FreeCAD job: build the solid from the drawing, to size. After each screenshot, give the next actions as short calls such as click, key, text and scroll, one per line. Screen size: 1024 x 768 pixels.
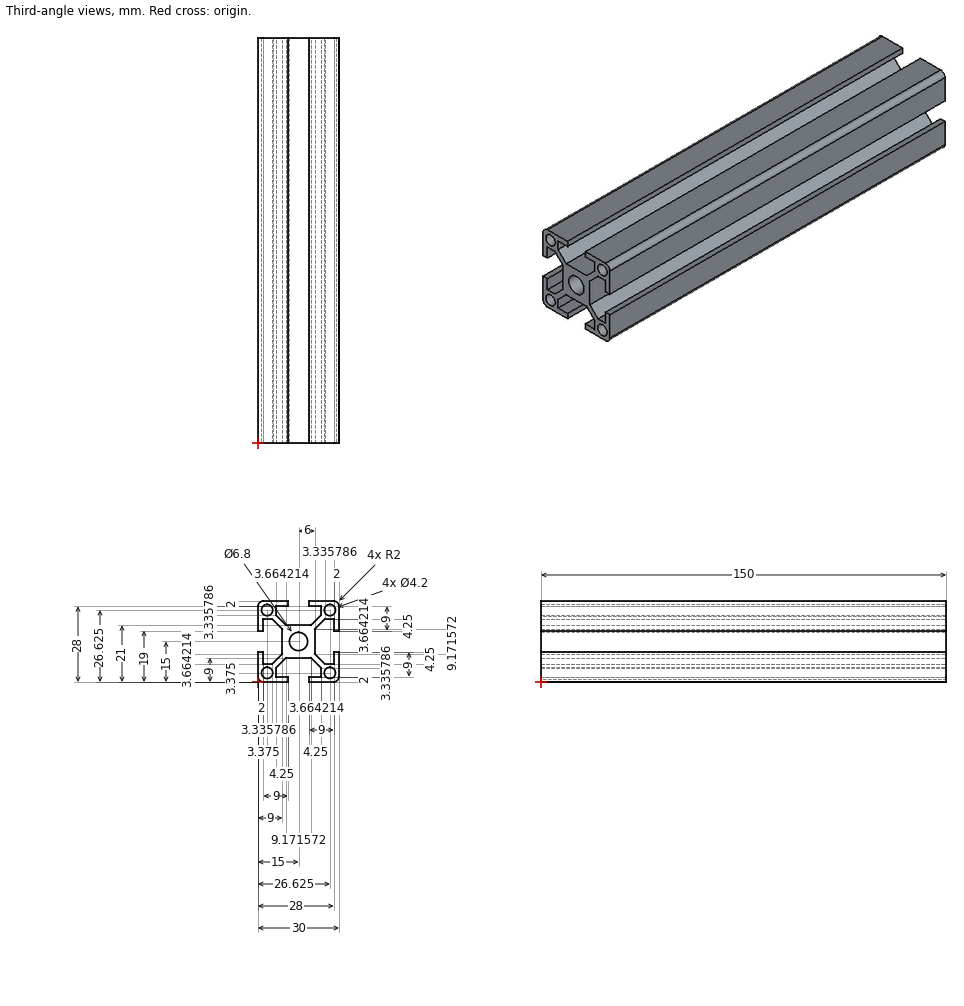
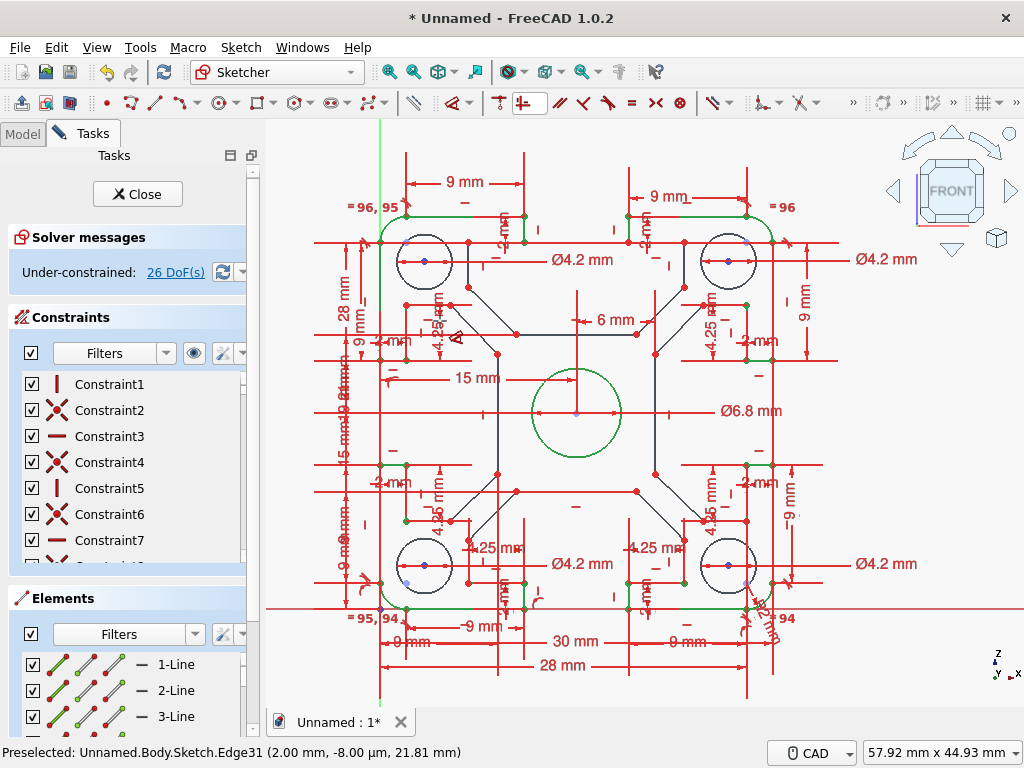
click(507, 243)
click(496, 277)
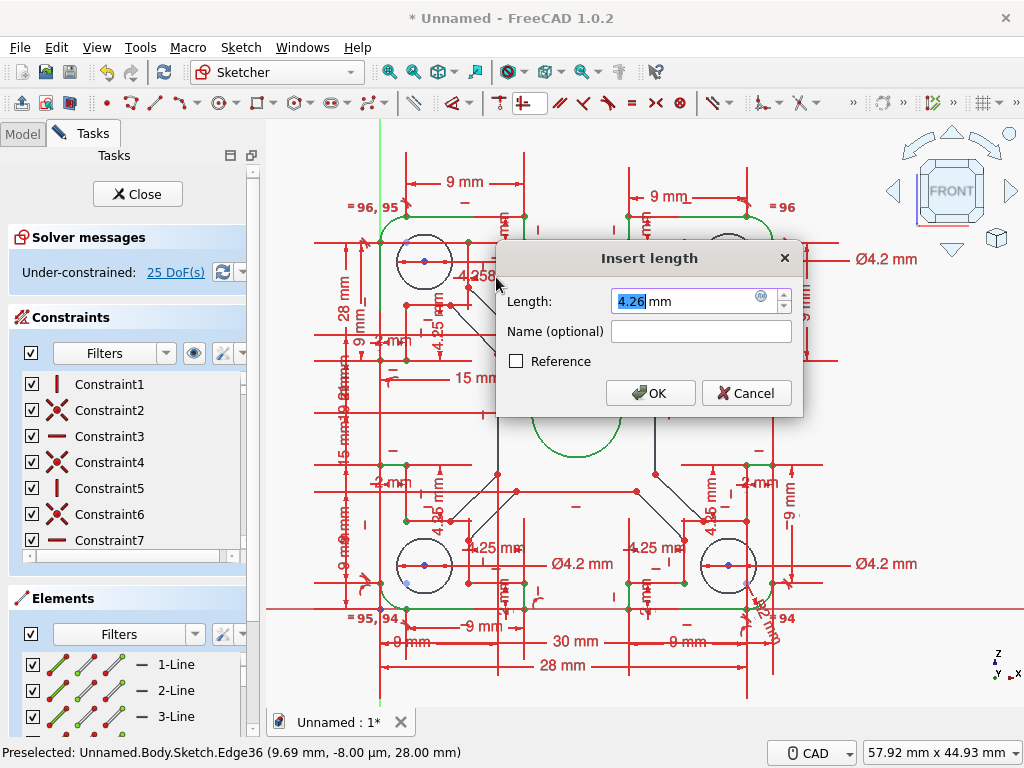
text(4.25)
key(Return)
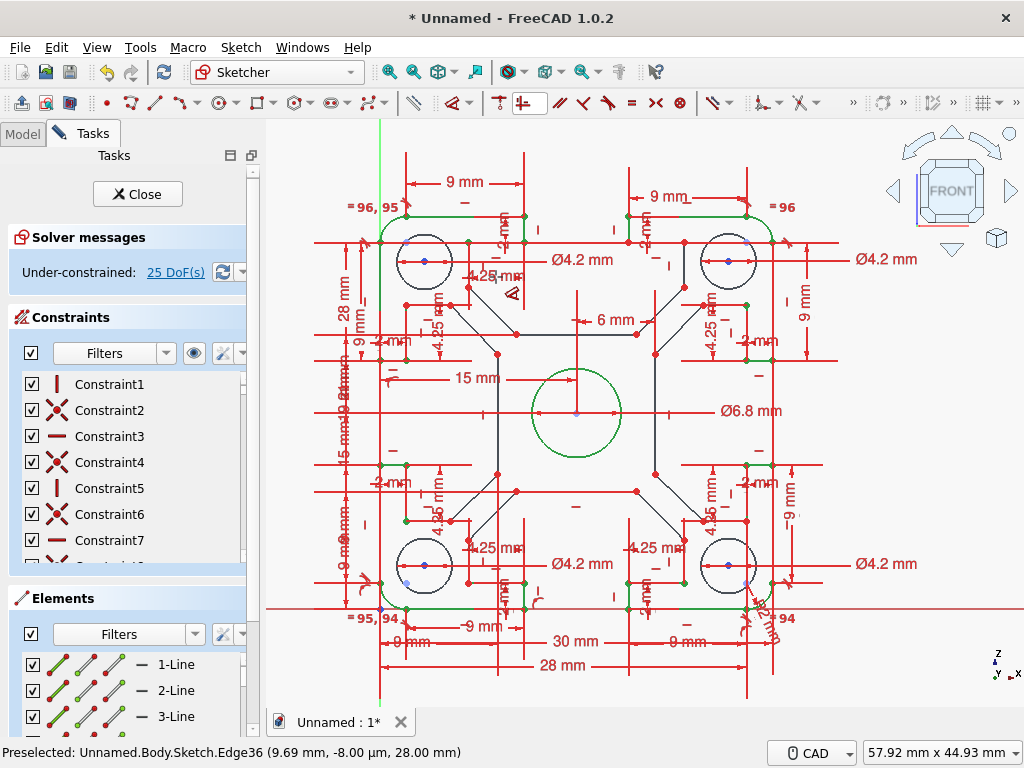
click(668, 243)
click(657, 277)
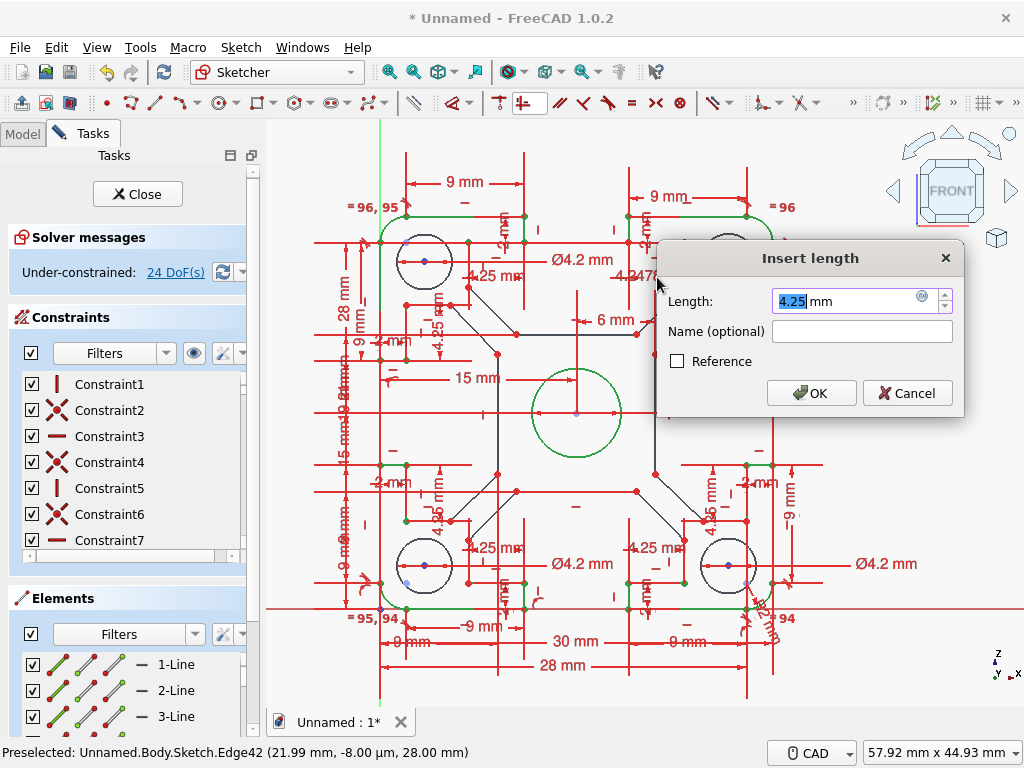
text(4.25)
key(Return)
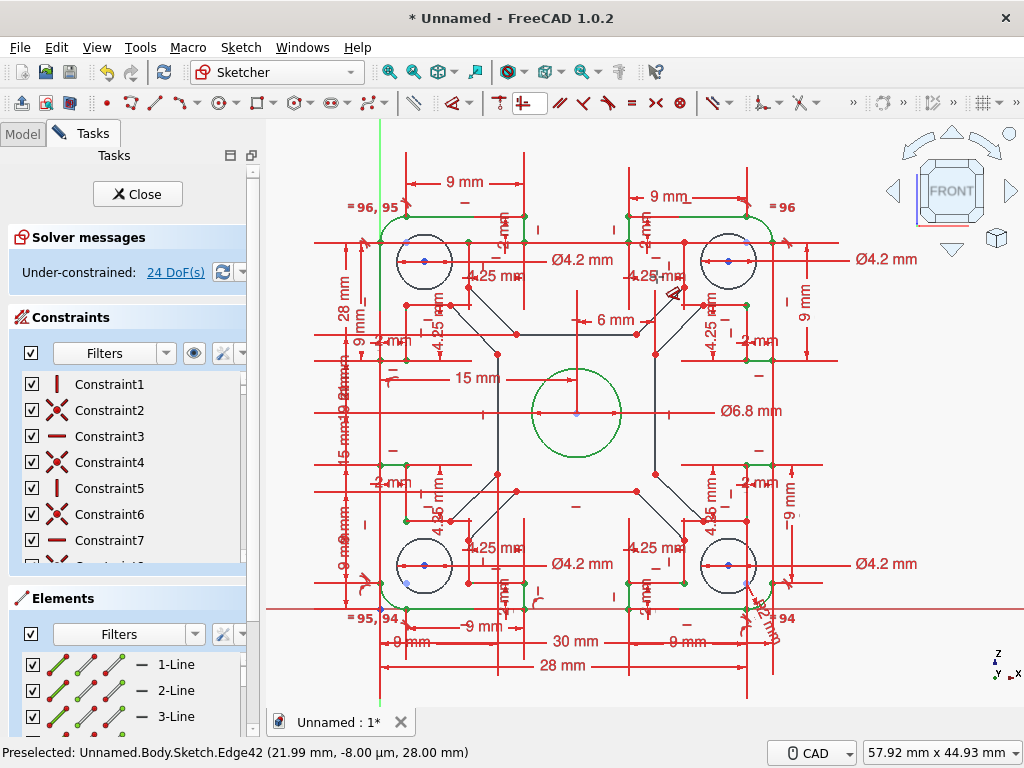
click(425, 262)
click(402, 667)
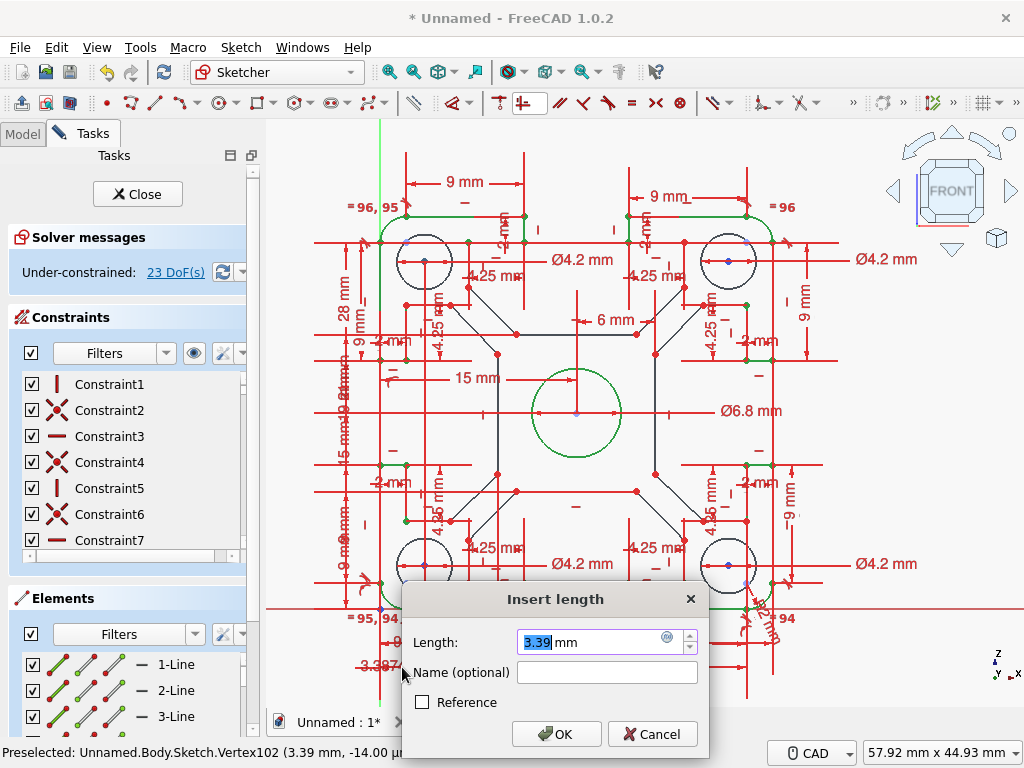
text(3.375)
key(Return)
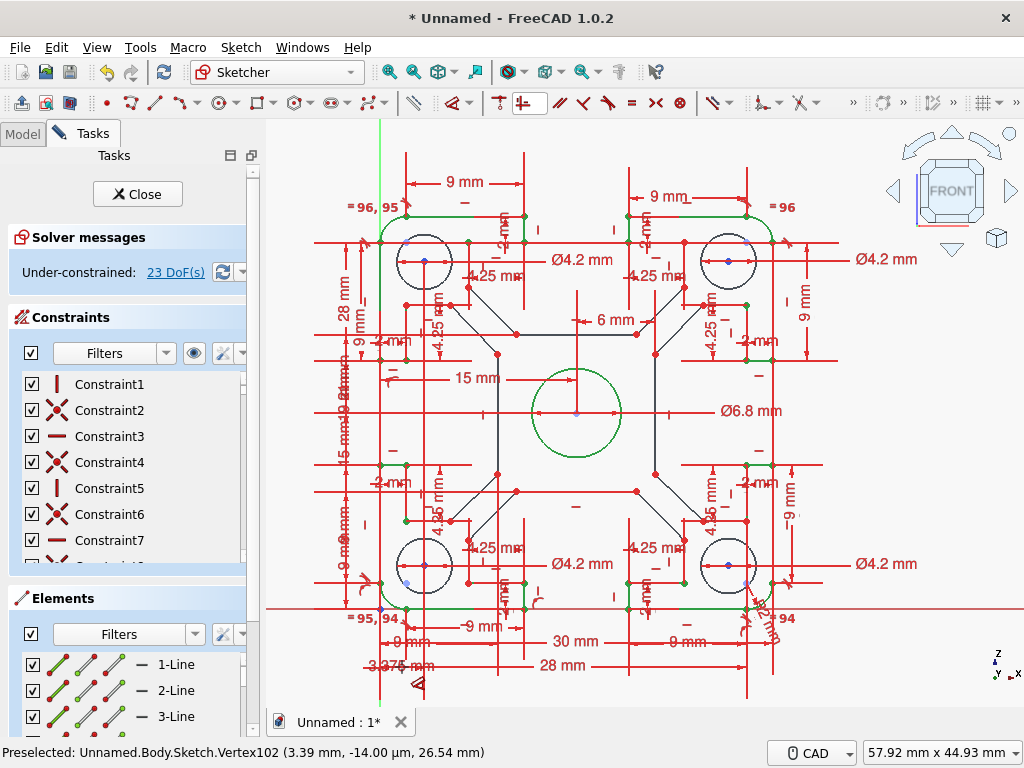
click(729, 566)
click(346, 588)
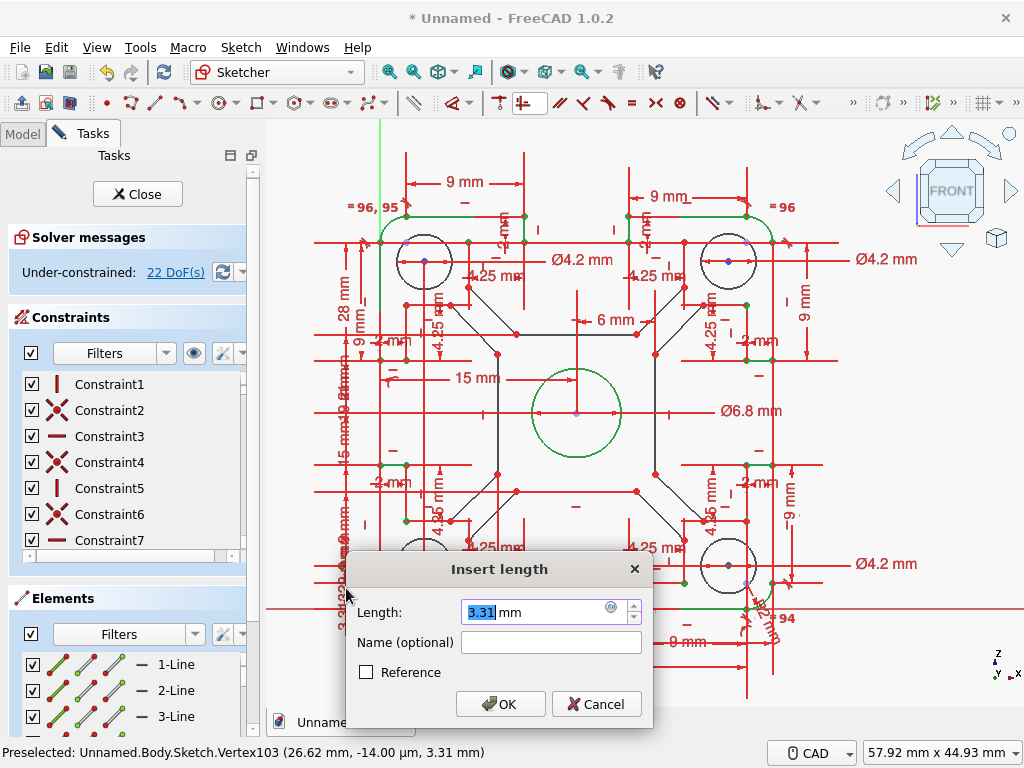
text(3.375)
key(Return)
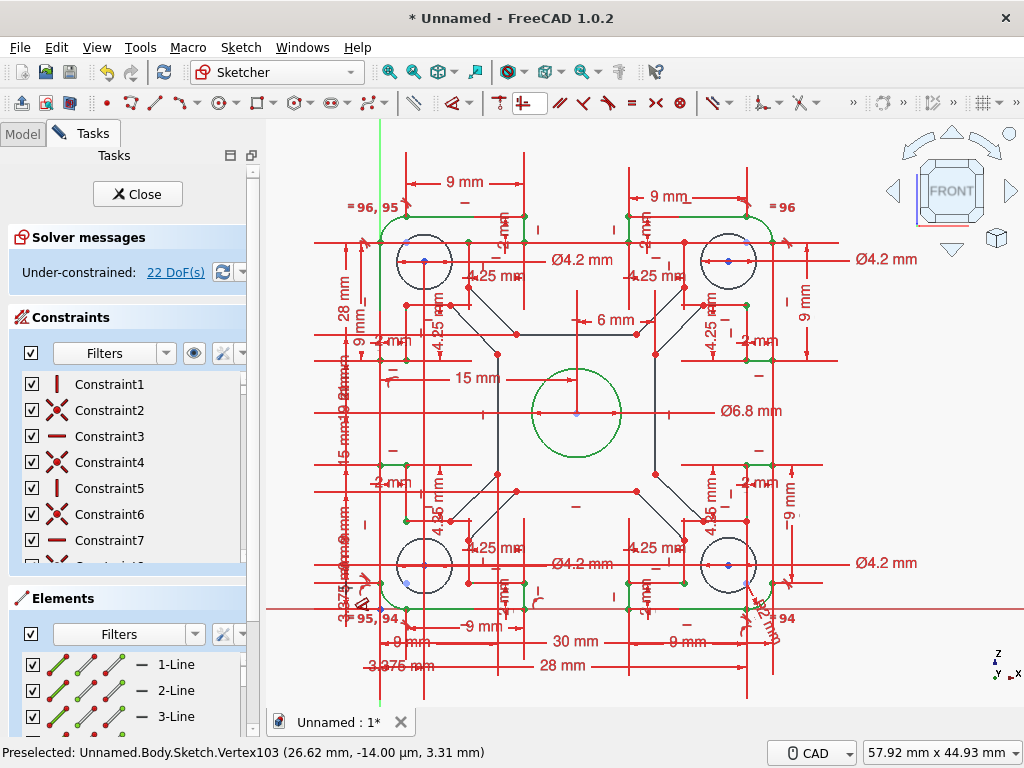
click(425, 566)
click(418, 436)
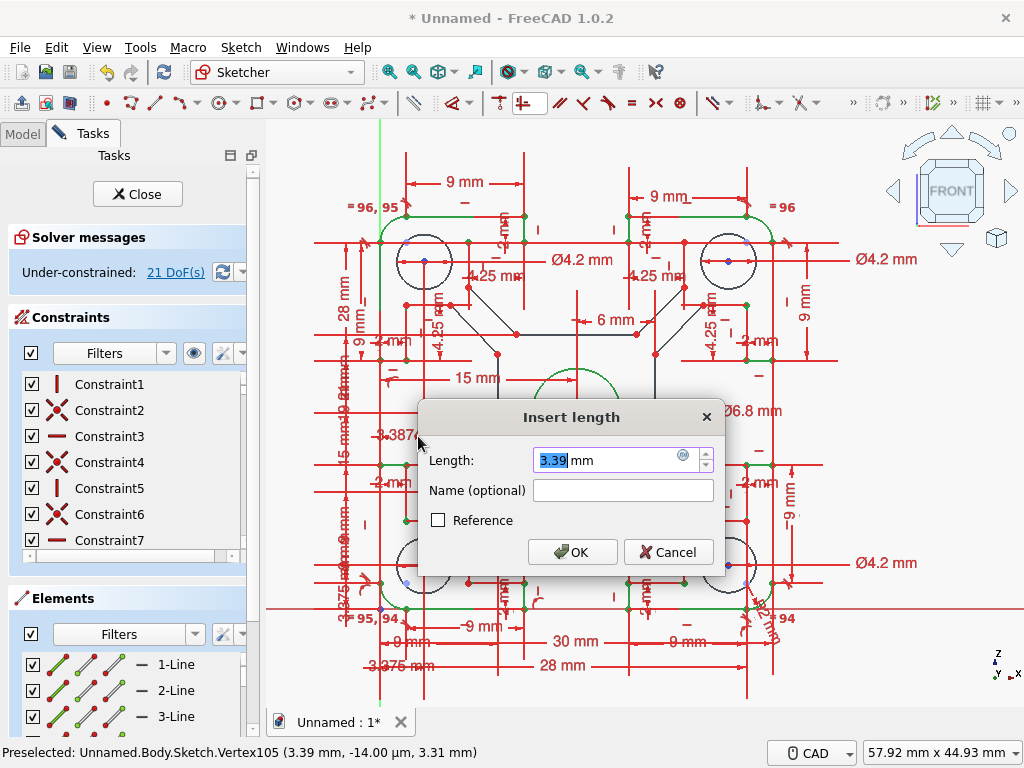
text(3.375)
key(Return)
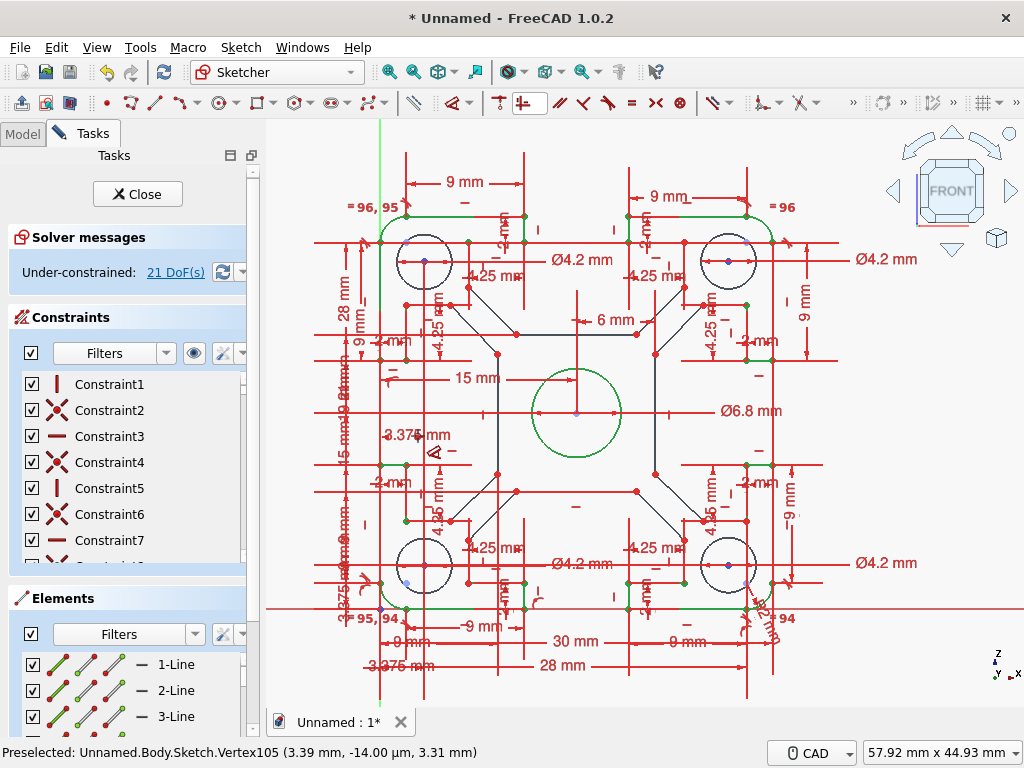
click(424, 566)
click(554, 573)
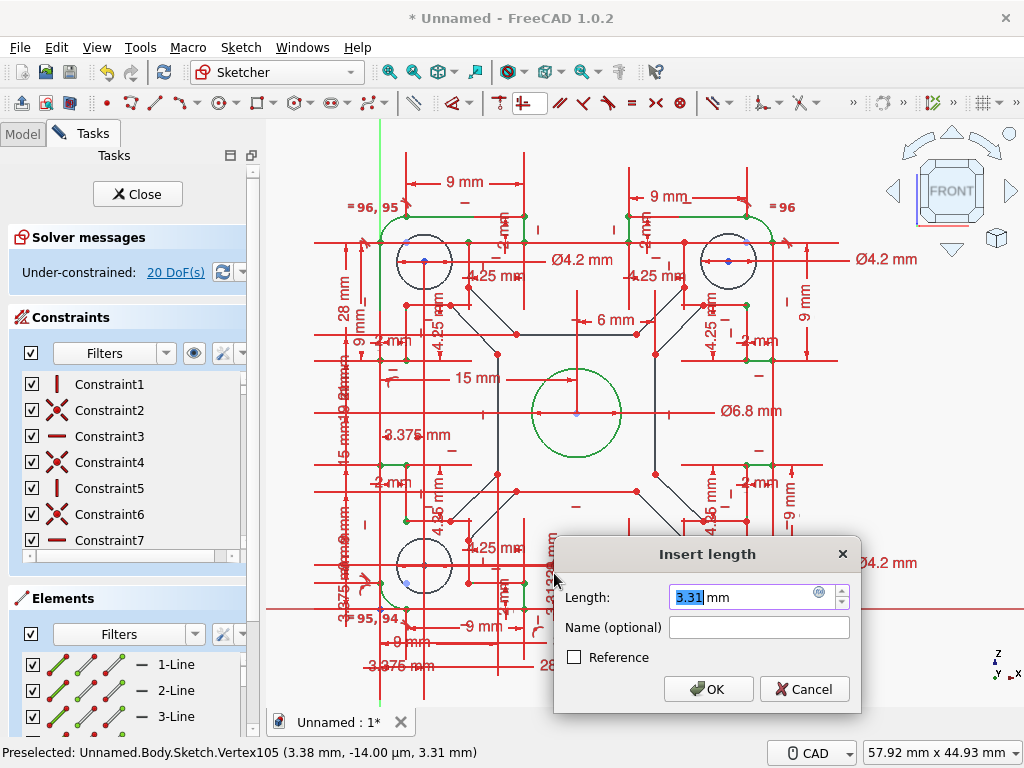
text(3.375)
key(Return)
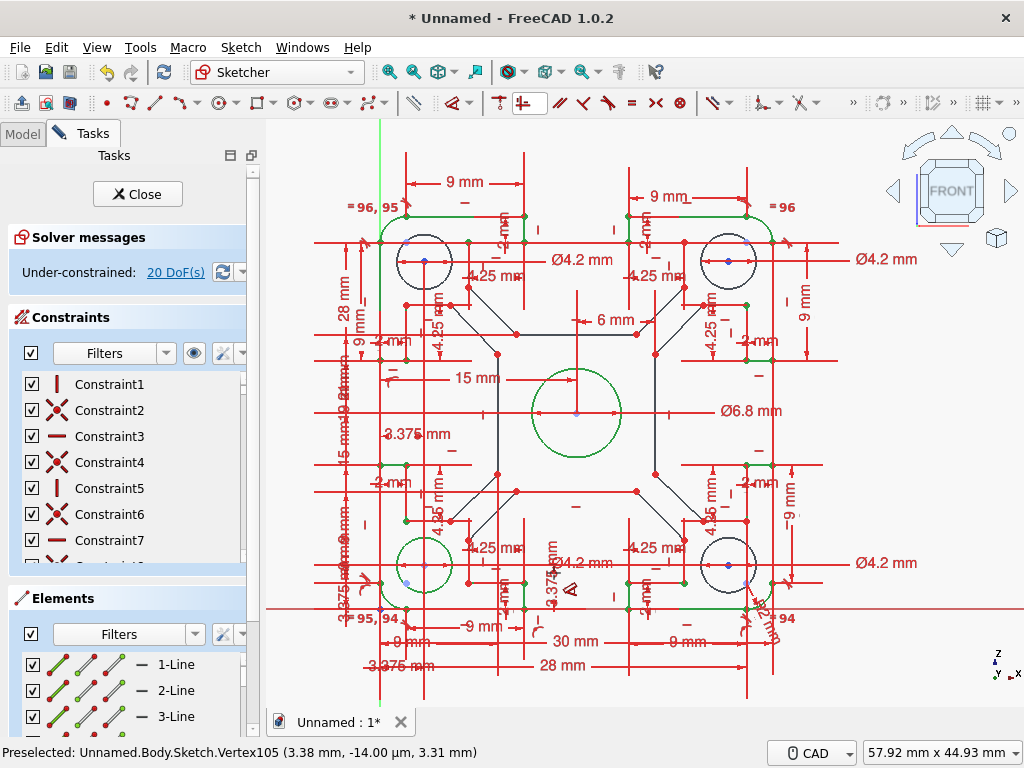
click(729, 261)
click(474, 667)